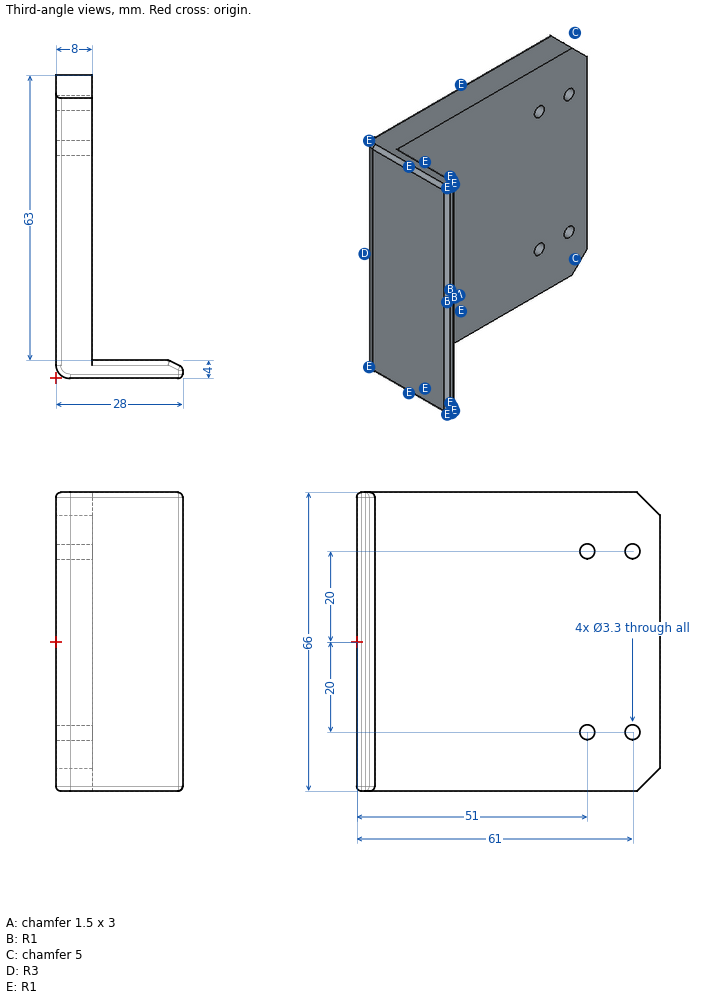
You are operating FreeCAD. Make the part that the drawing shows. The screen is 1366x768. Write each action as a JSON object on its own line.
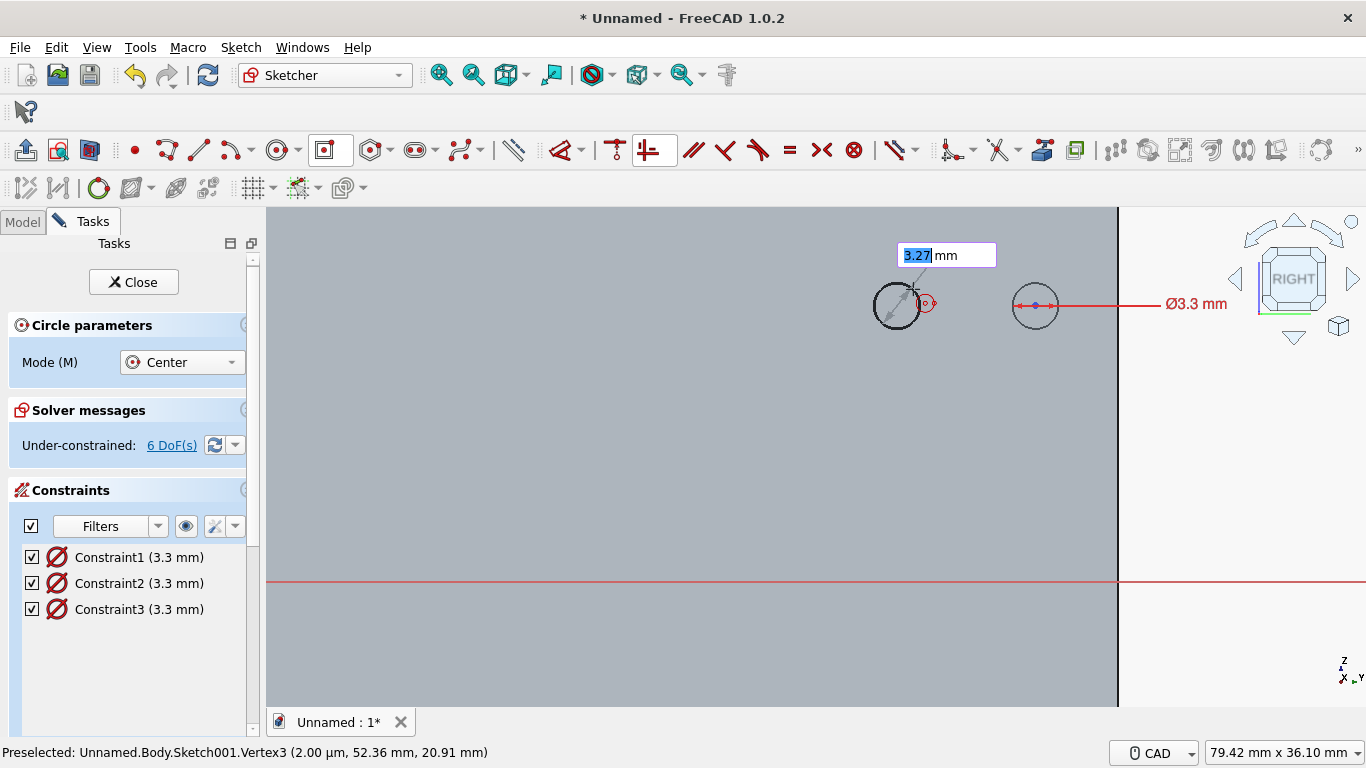
{"action": "type", "text": "3.3"}
{"action": "key", "text": "Return"}
{"action": "key", "text": "Escape"}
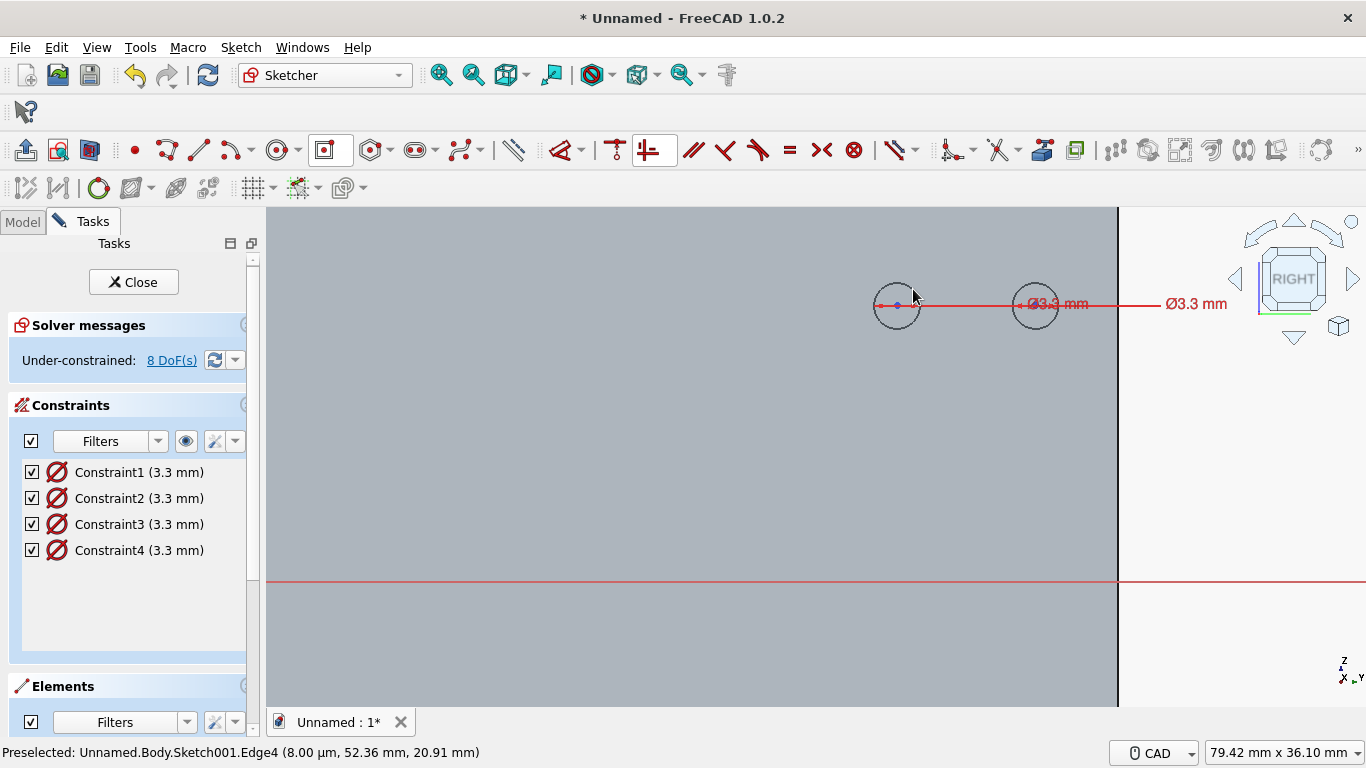
{"action": "scroll", "coordinate": [898, 305], "scroll_direction": "down", "scroll_amount": 3}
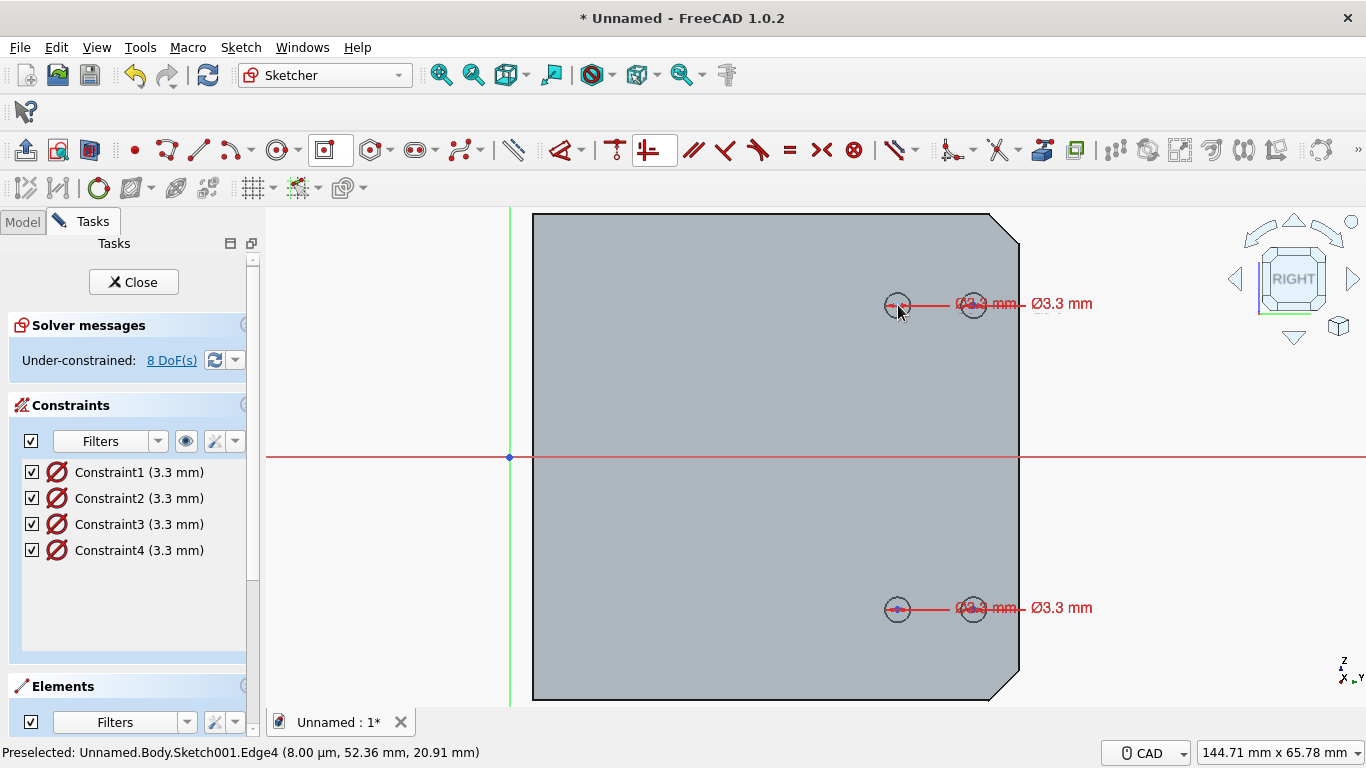
{"action": "left_click", "coordinate": [974, 610]}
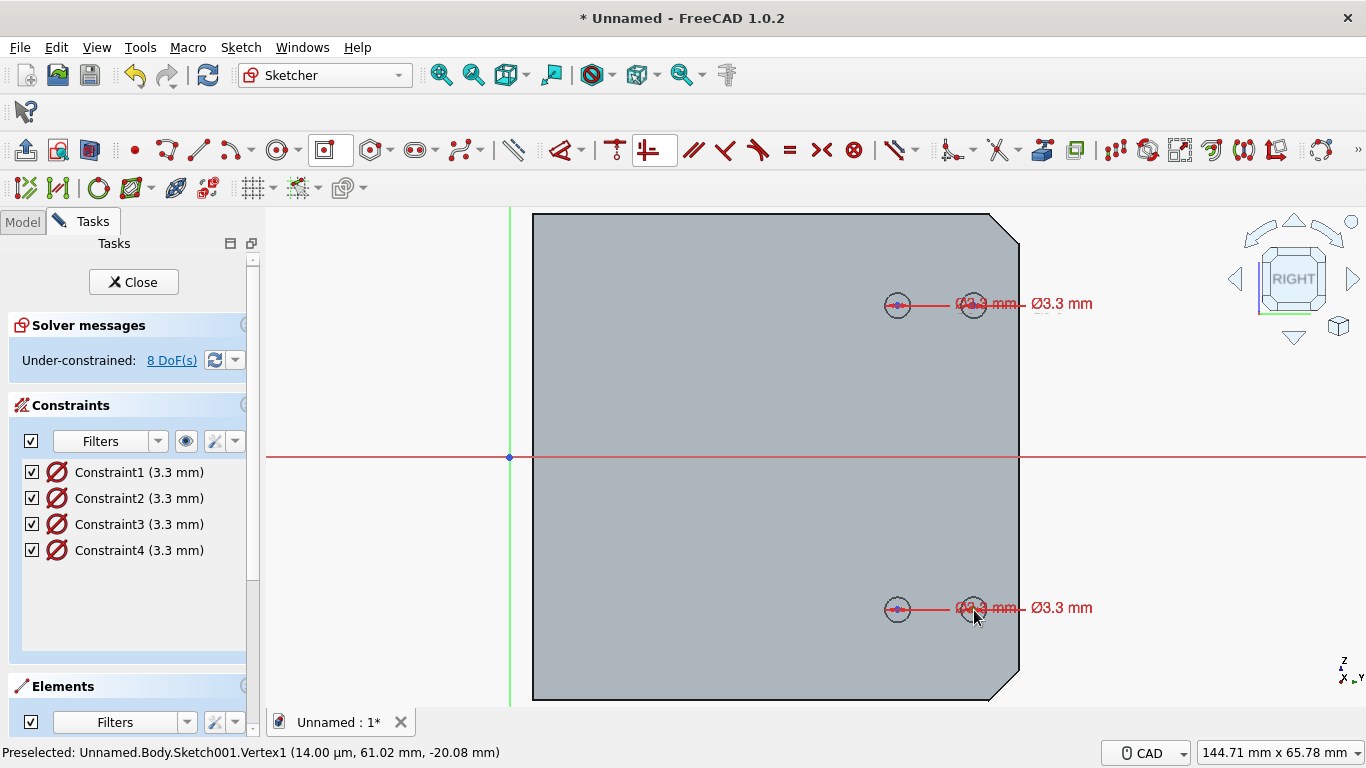
{"action": "left_click", "coordinate": [974, 306]}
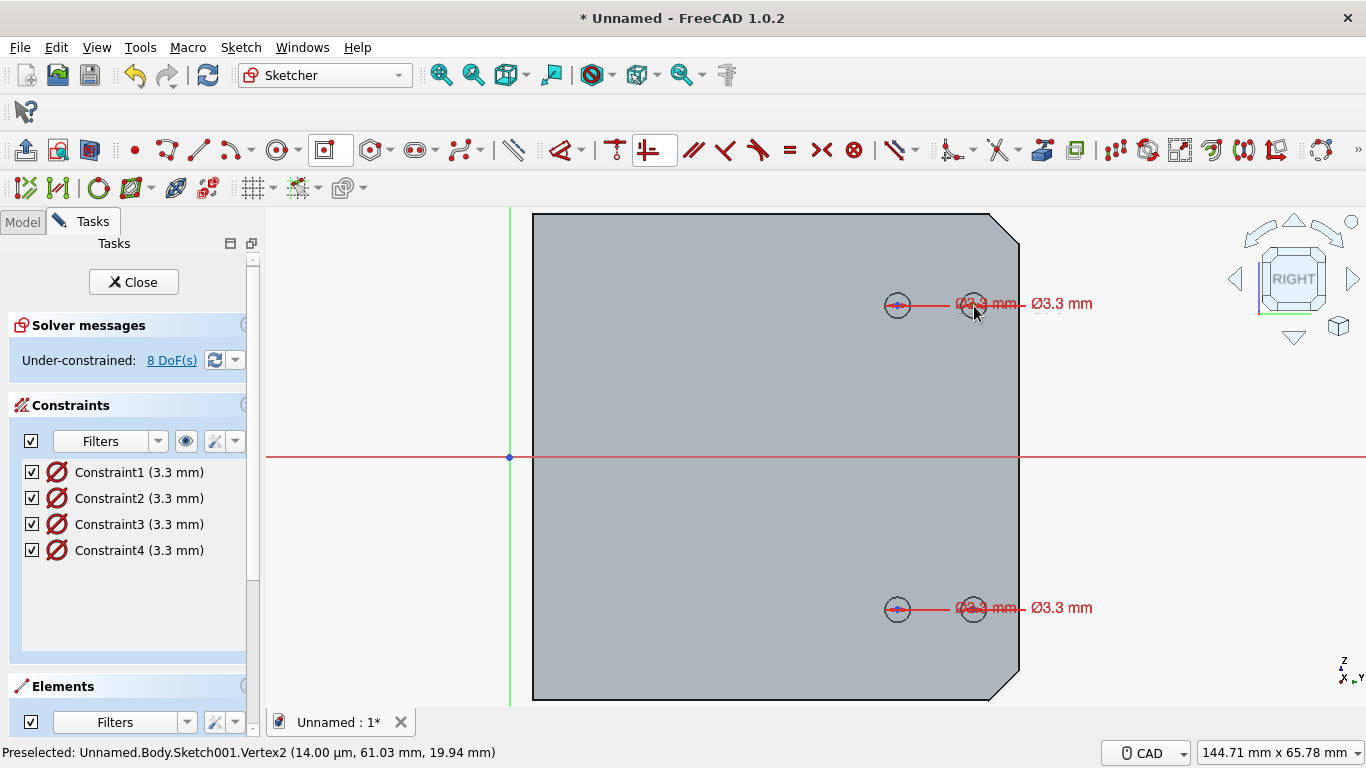
{"action": "key", "text": "v"}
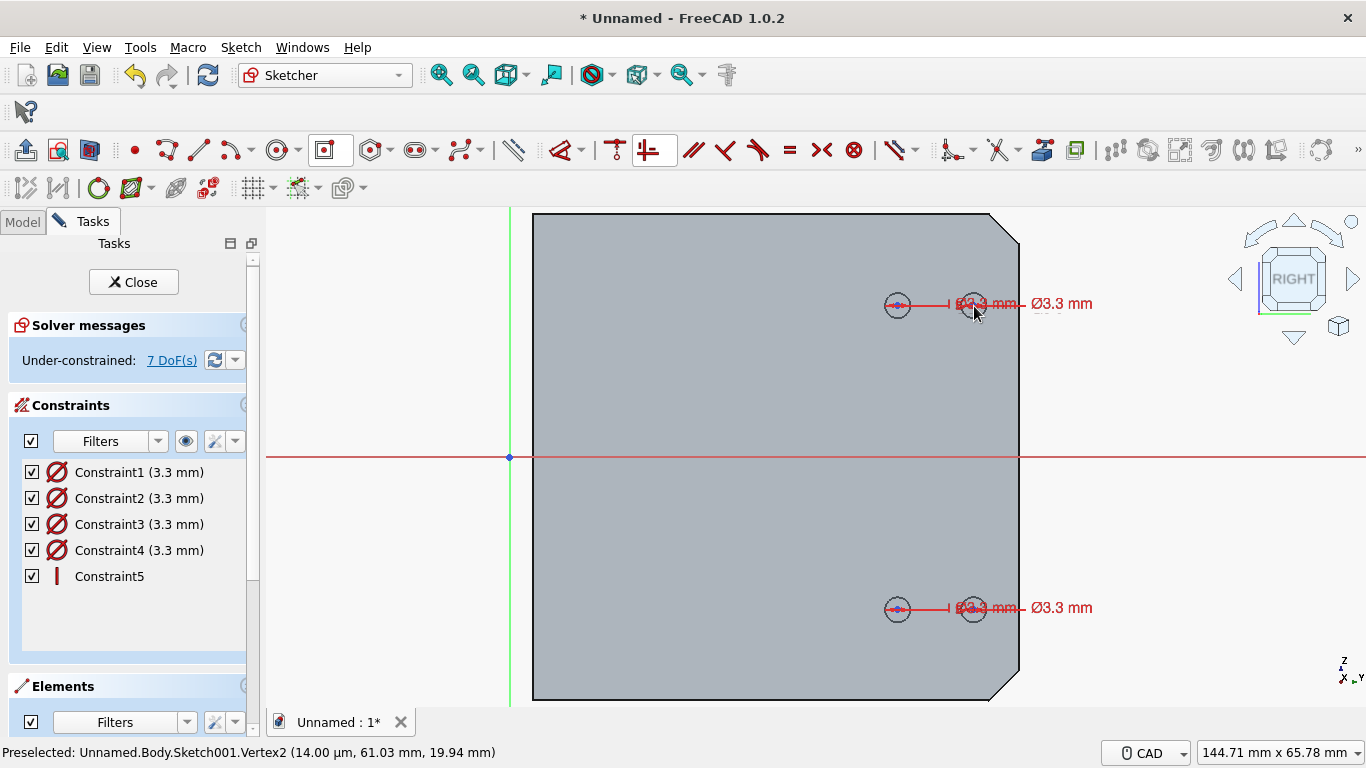
{"action": "left_click", "coordinate": [974, 610]}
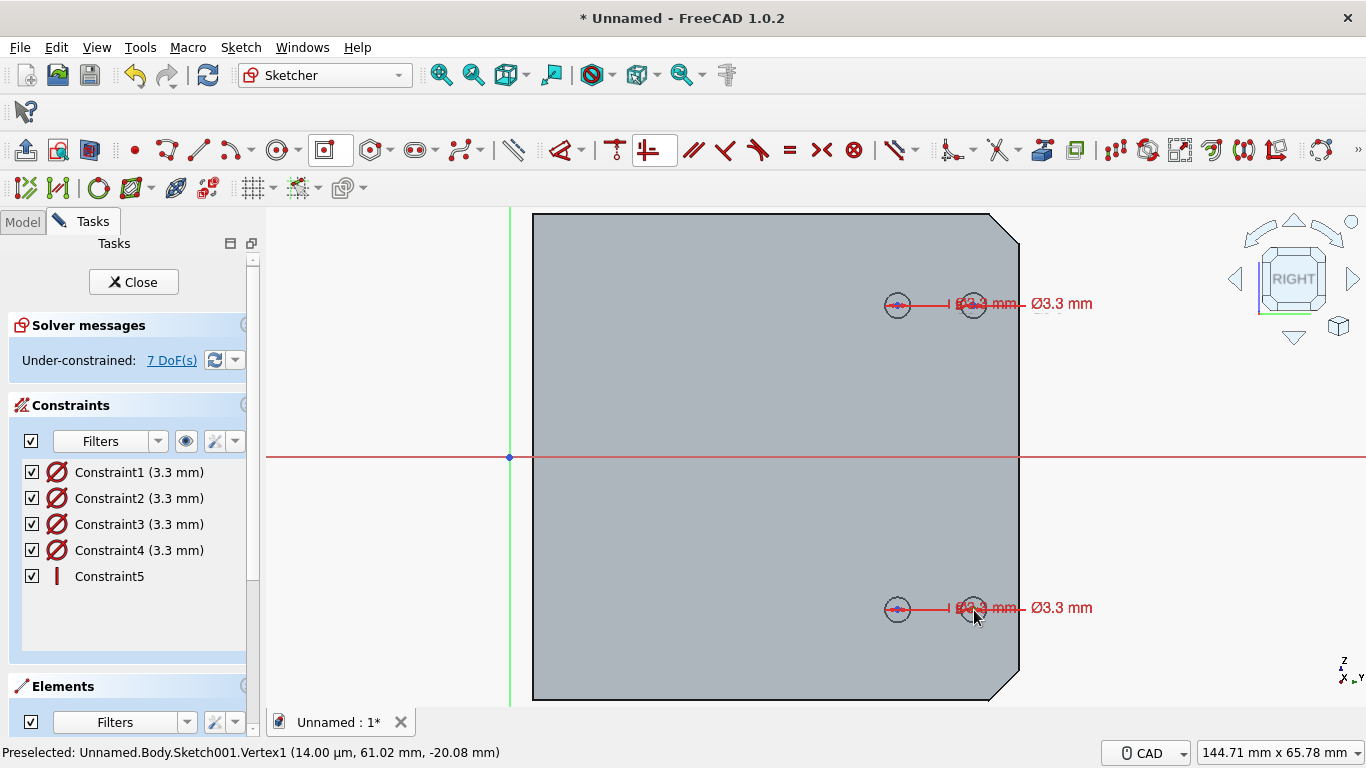
{"action": "left_click", "coordinate": [898, 610]}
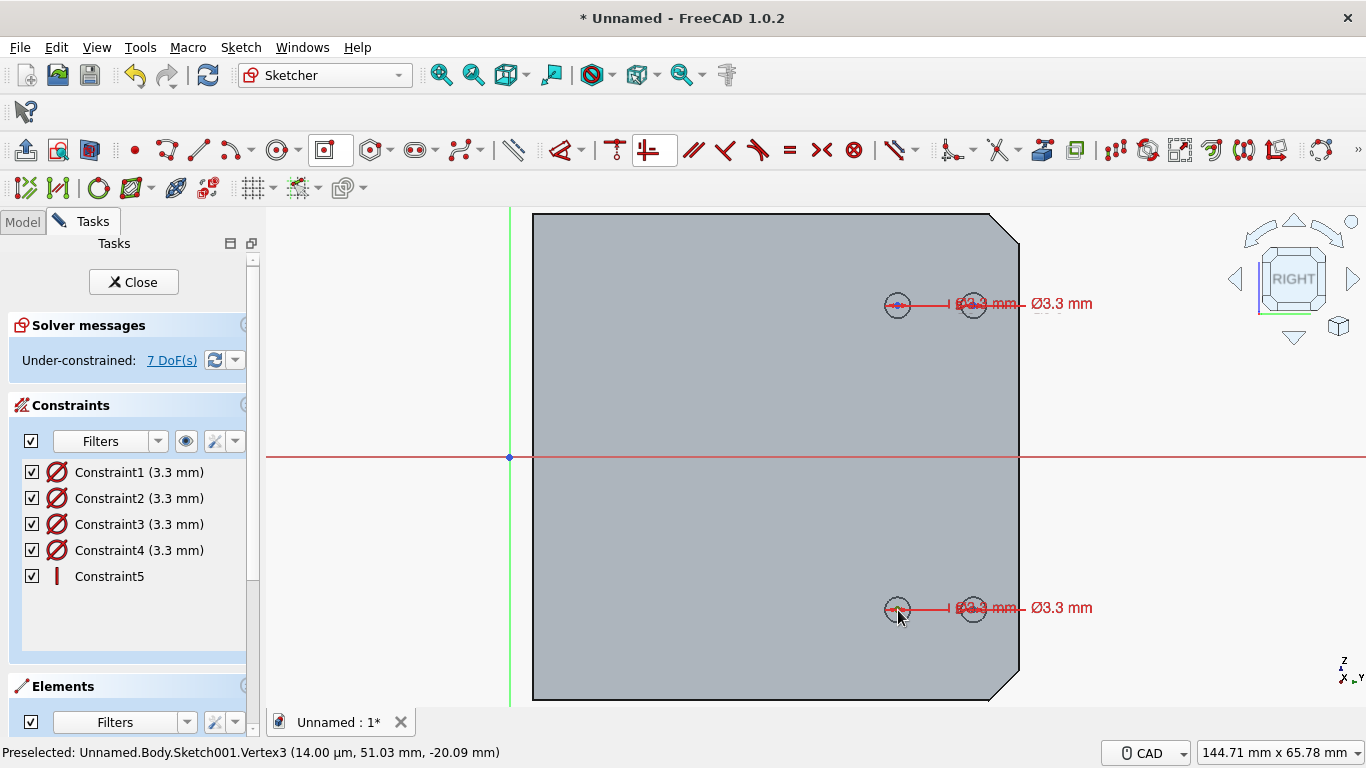
{"action": "left_click", "coordinate": [672, 150]}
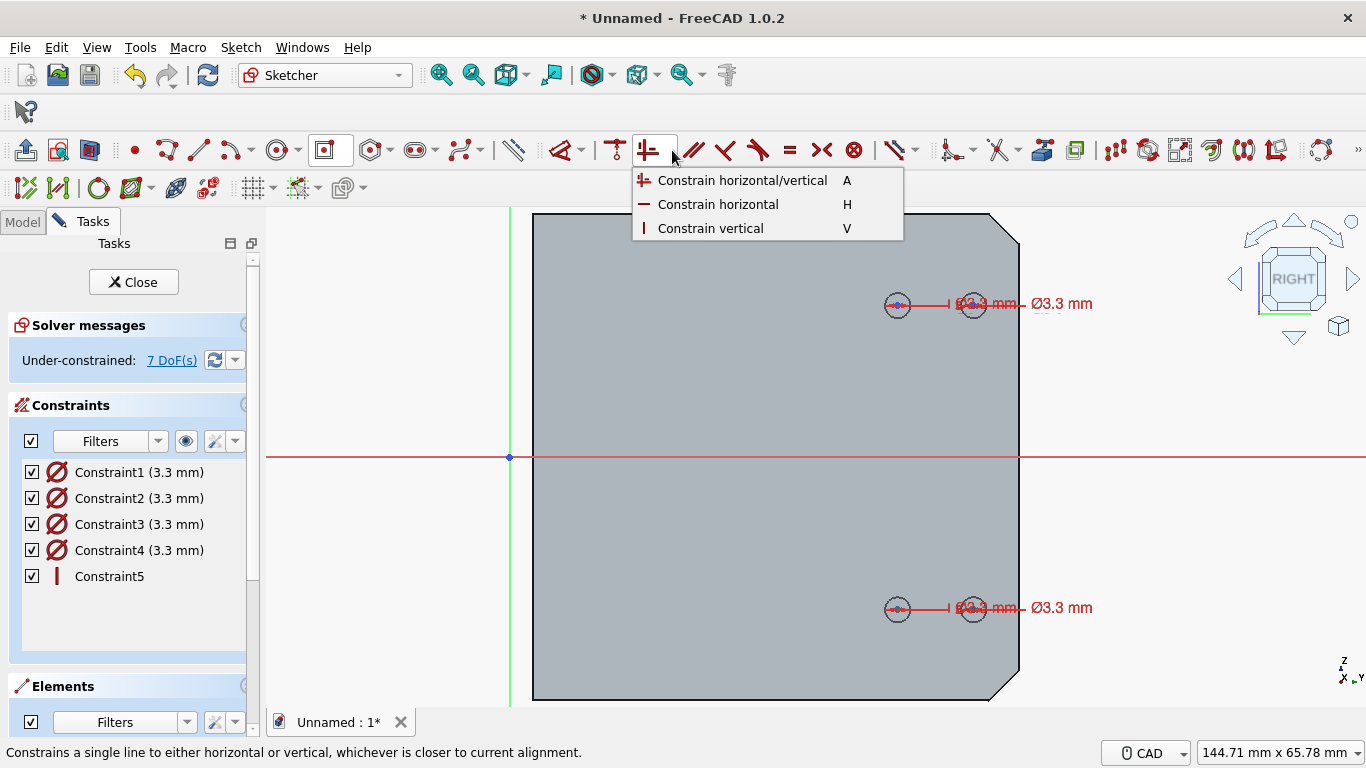
{"action": "left_click", "coordinate": [768, 204]}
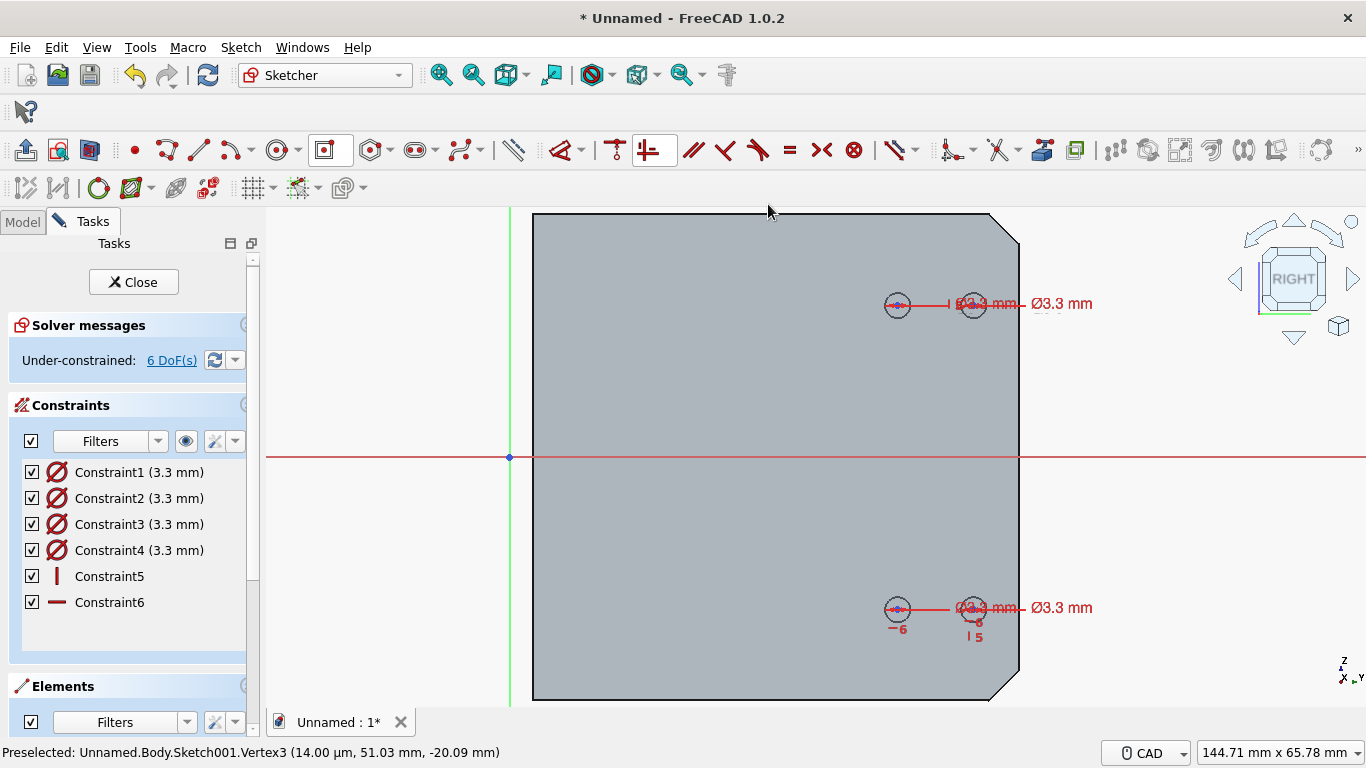
{"action": "left_click", "coordinate": [898, 610]}